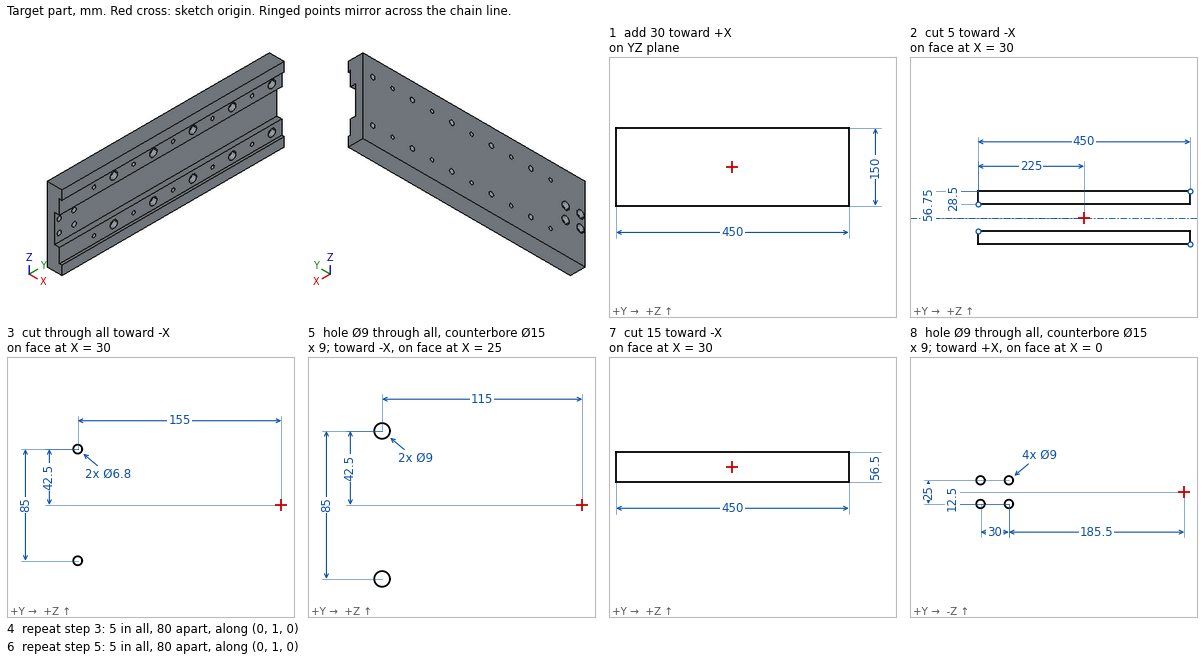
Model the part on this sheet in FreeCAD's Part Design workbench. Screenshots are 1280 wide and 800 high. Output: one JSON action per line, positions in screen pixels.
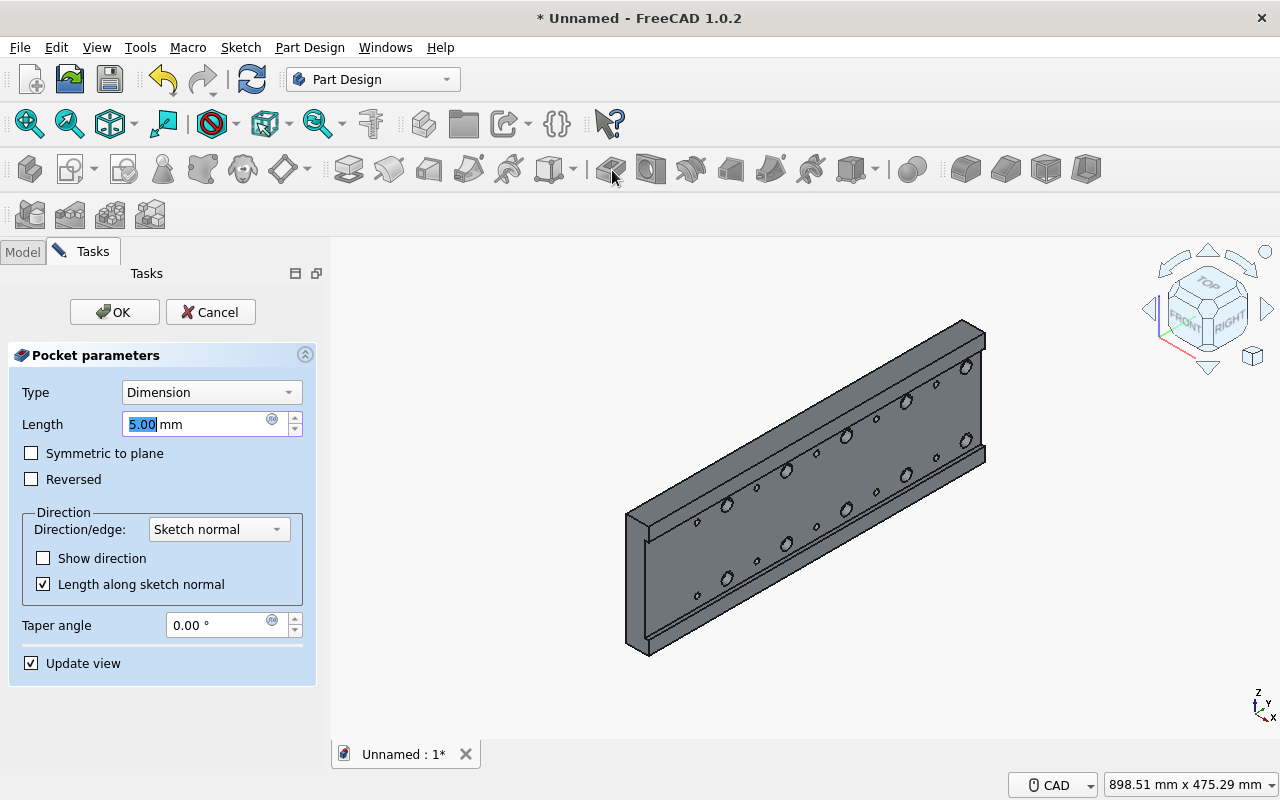
{"action": "type", "text": "15"}
{"action": "key", "text": "Tab"}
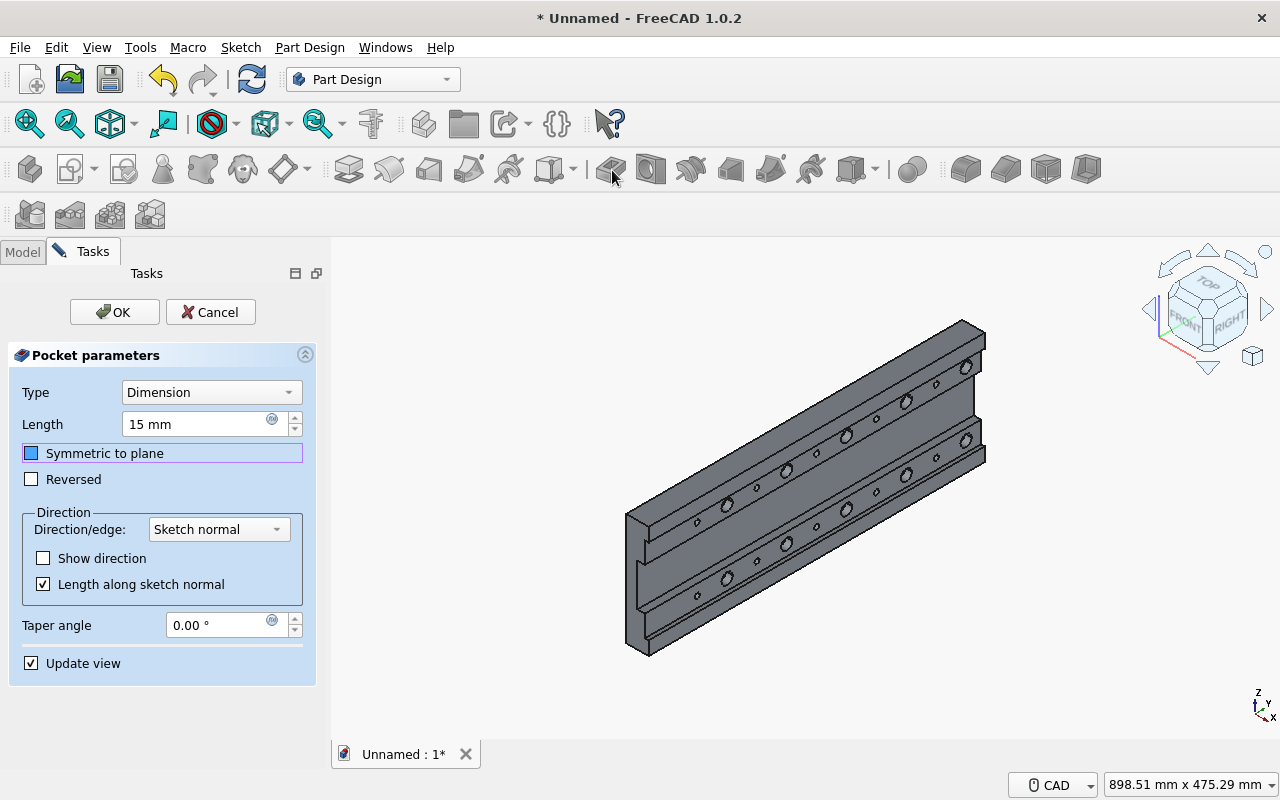
{"action": "left_click", "coordinate": [115, 312]}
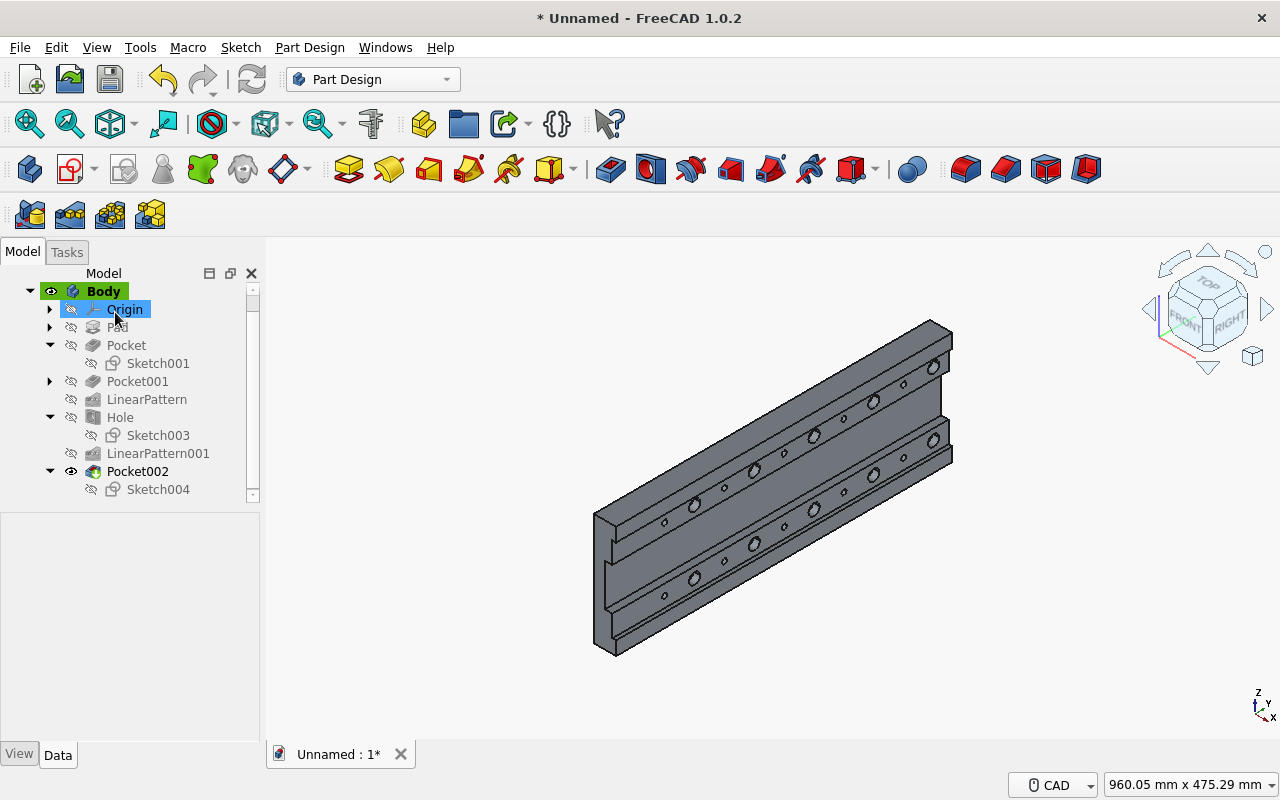
{"action": "key", "text": "6"}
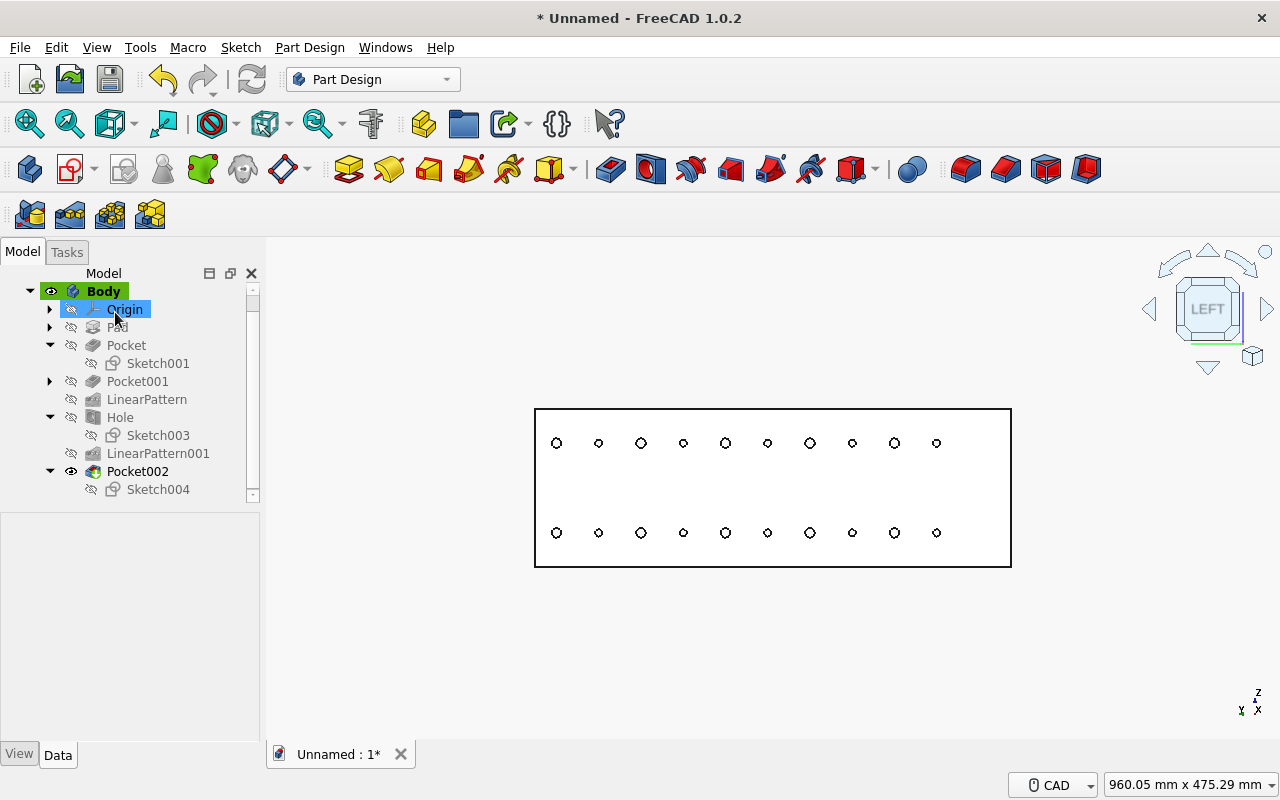
{"action": "left_click", "coordinate": [705, 487]}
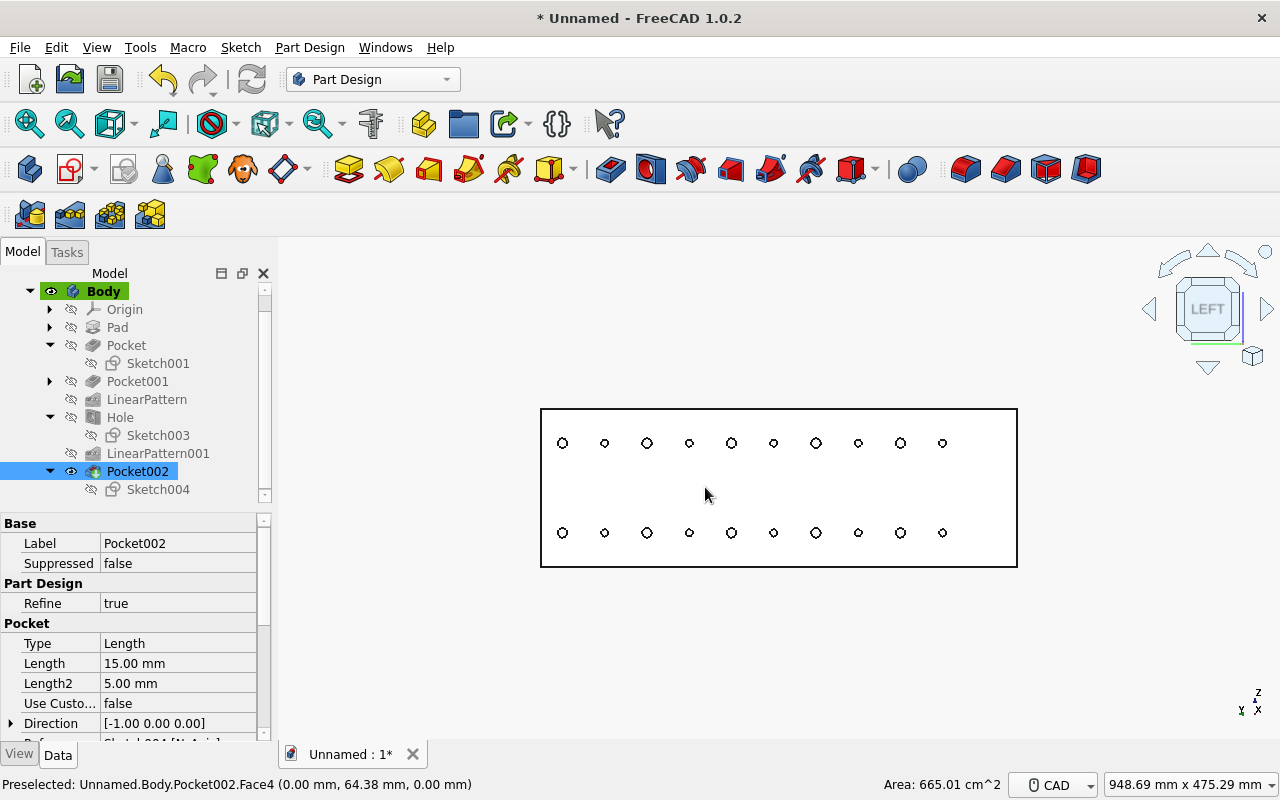
{"action": "left_click", "coordinate": [70, 170]}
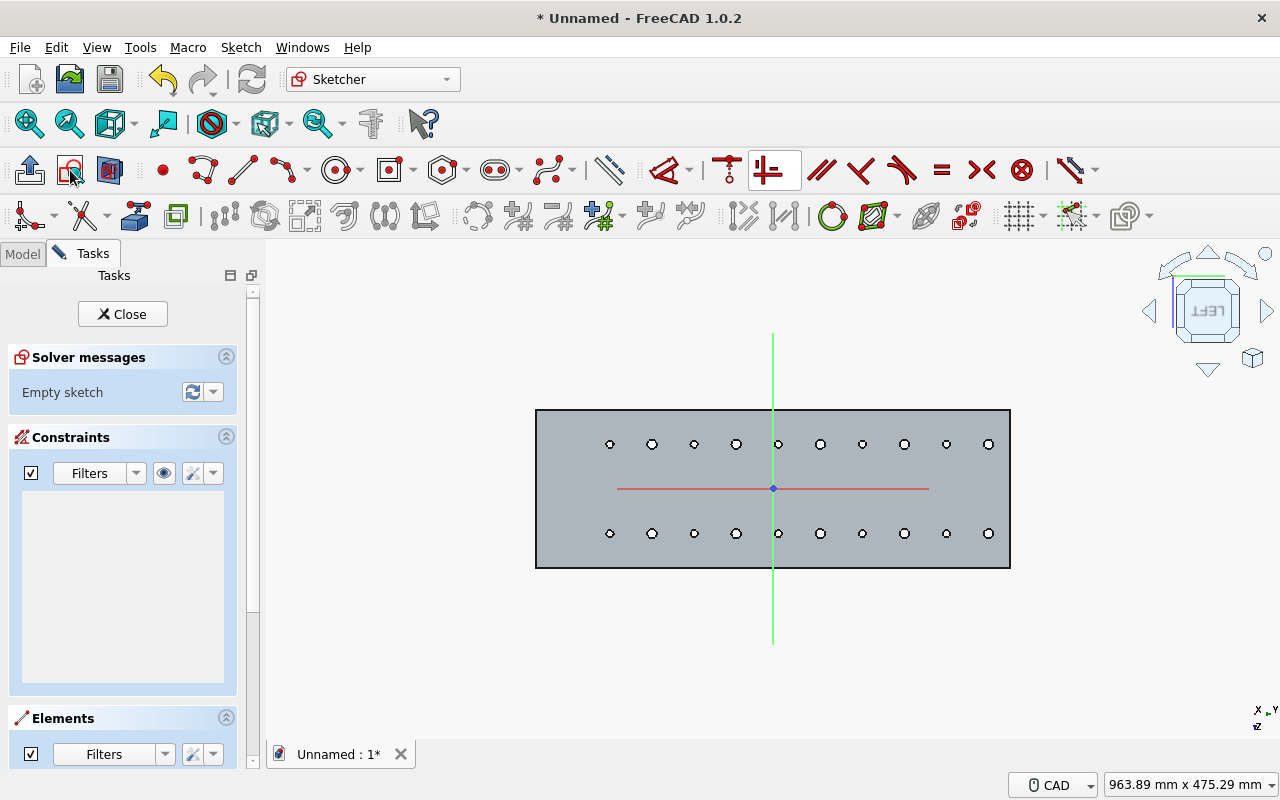
{"action": "scroll", "coordinate": [544, 489], "scroll_direction": "up", "scroll_amount": 11}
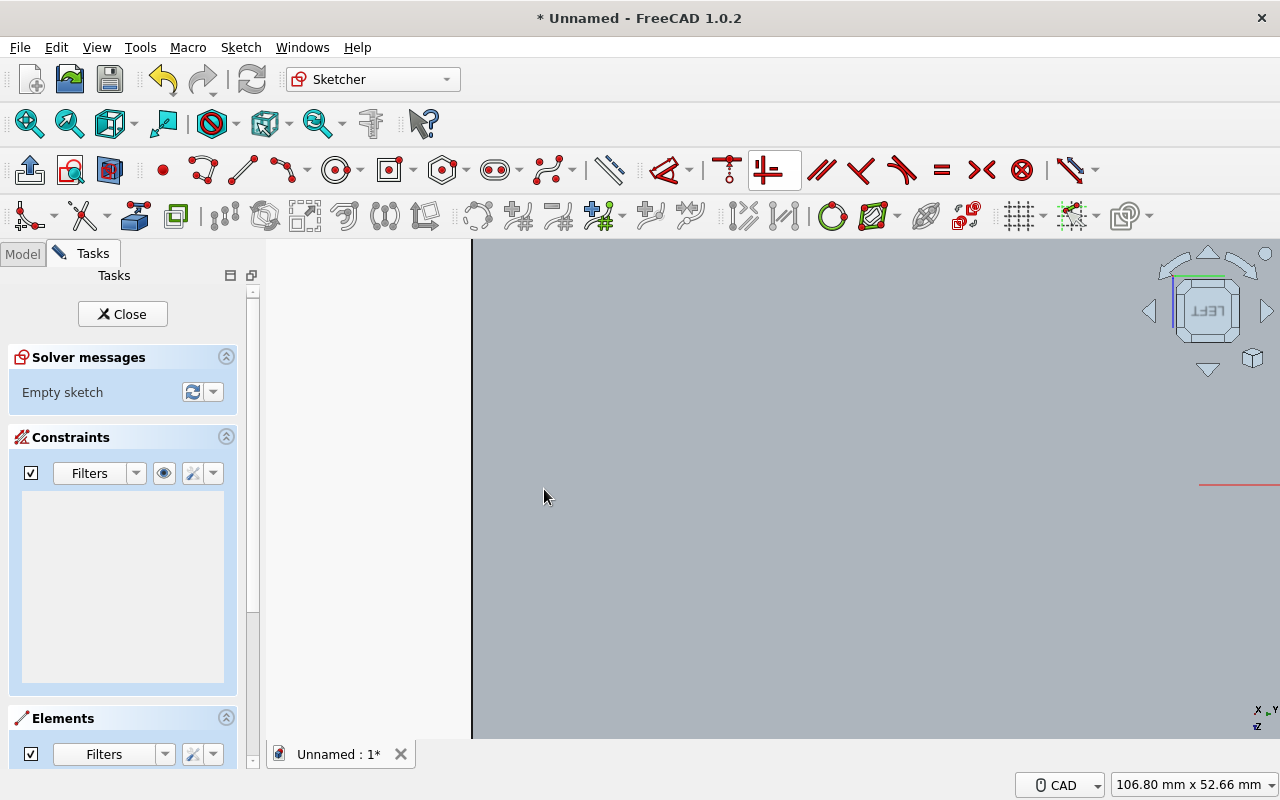
{"action": "left_click", "coordinate": [336, 170]}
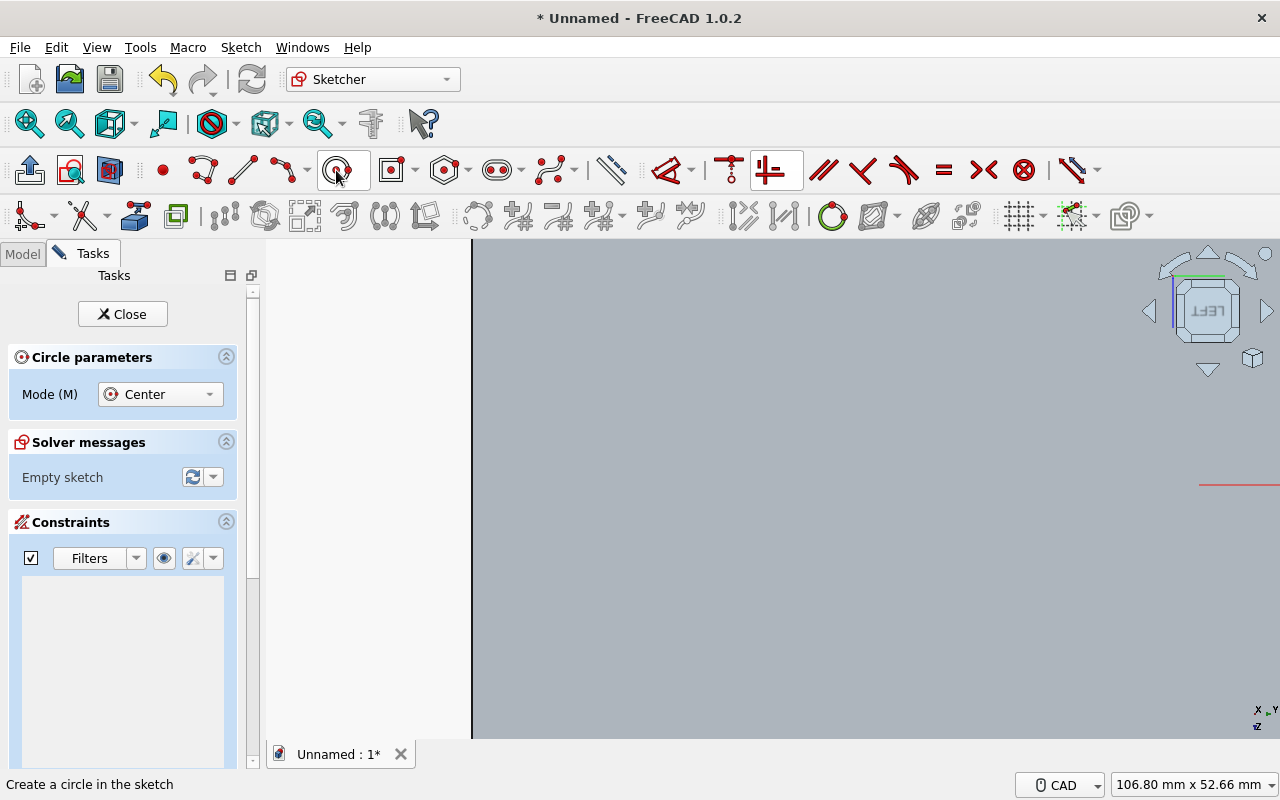
{"action": "left_click", "coordinate": [847, 604]}
{"action": "left_click", "coordinate": [878, 573]}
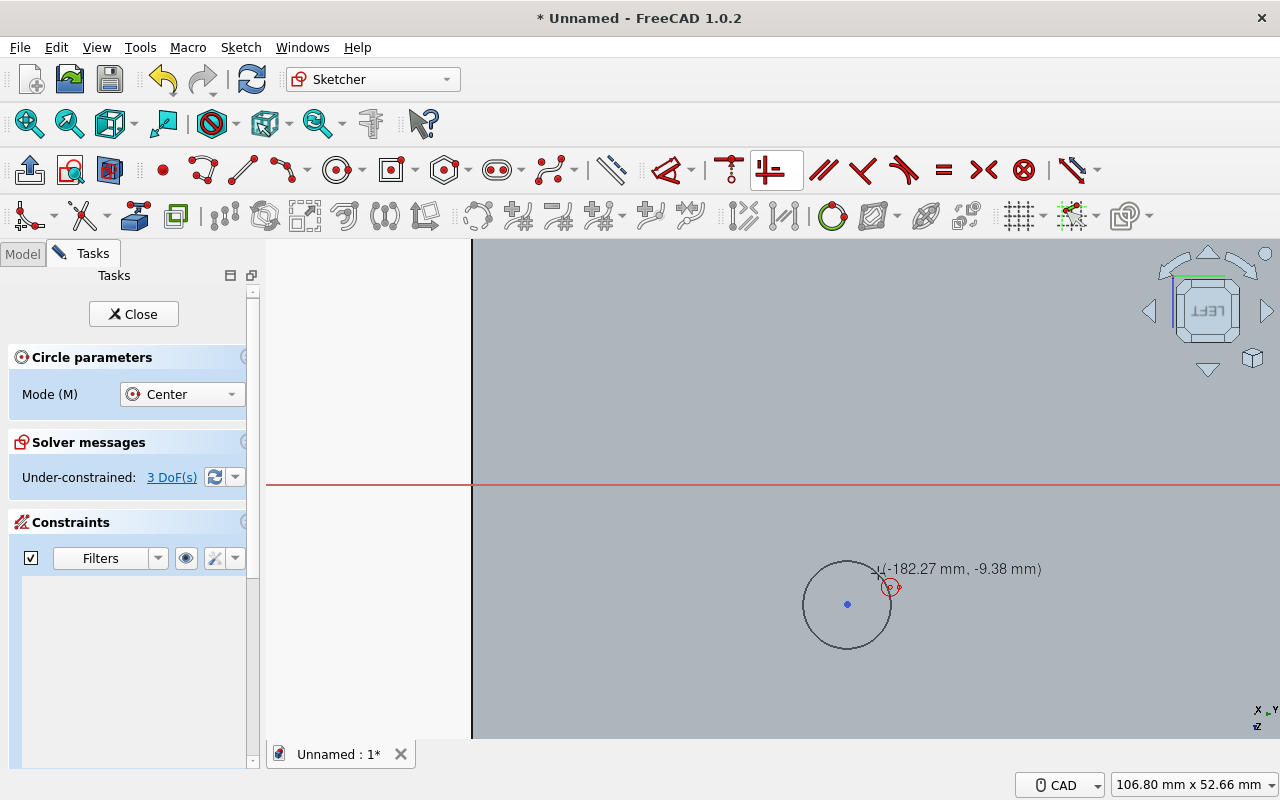
{"action": "left_click", "coordinate": [847, 366]}
{"action": "left_click", "coordinate": [878, 336]}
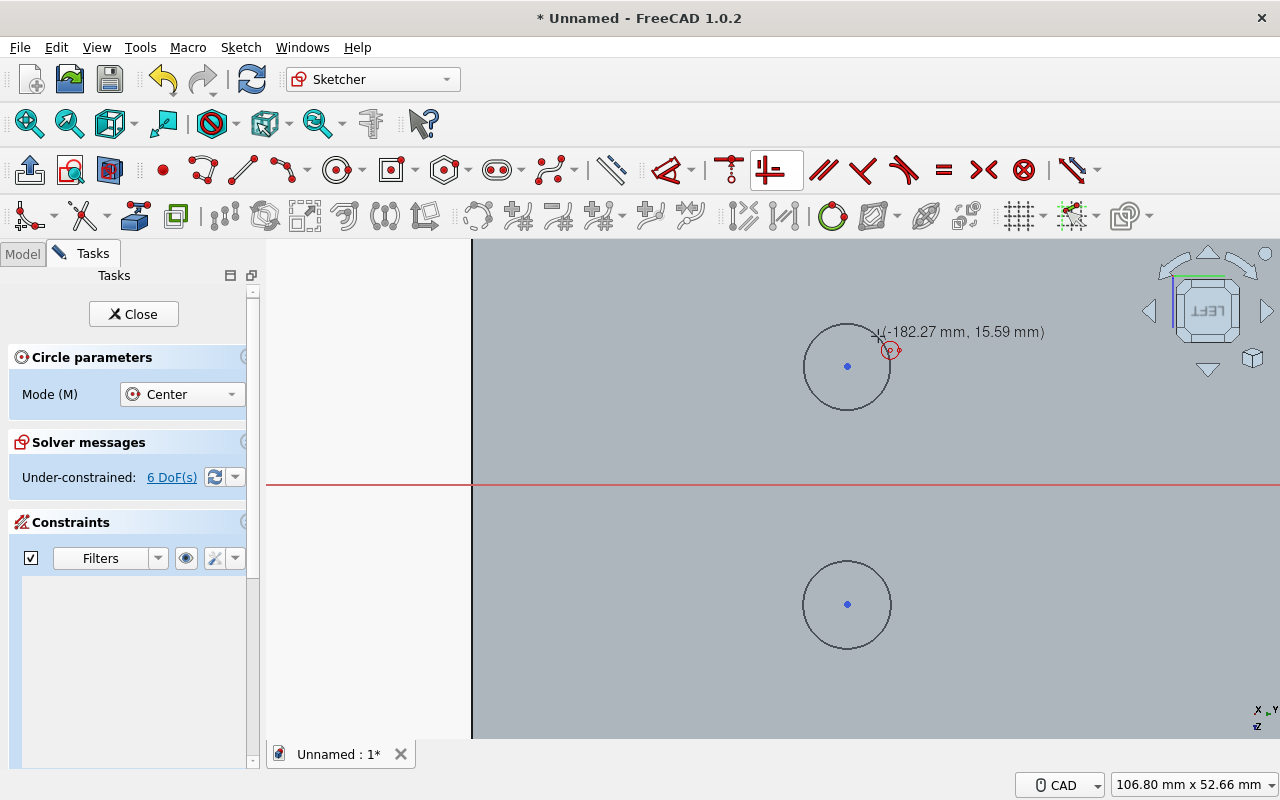
{"action": "left_click", "coordinate": [563, 604]}
{"action": "left_click", "coordinate": [593, 573]}